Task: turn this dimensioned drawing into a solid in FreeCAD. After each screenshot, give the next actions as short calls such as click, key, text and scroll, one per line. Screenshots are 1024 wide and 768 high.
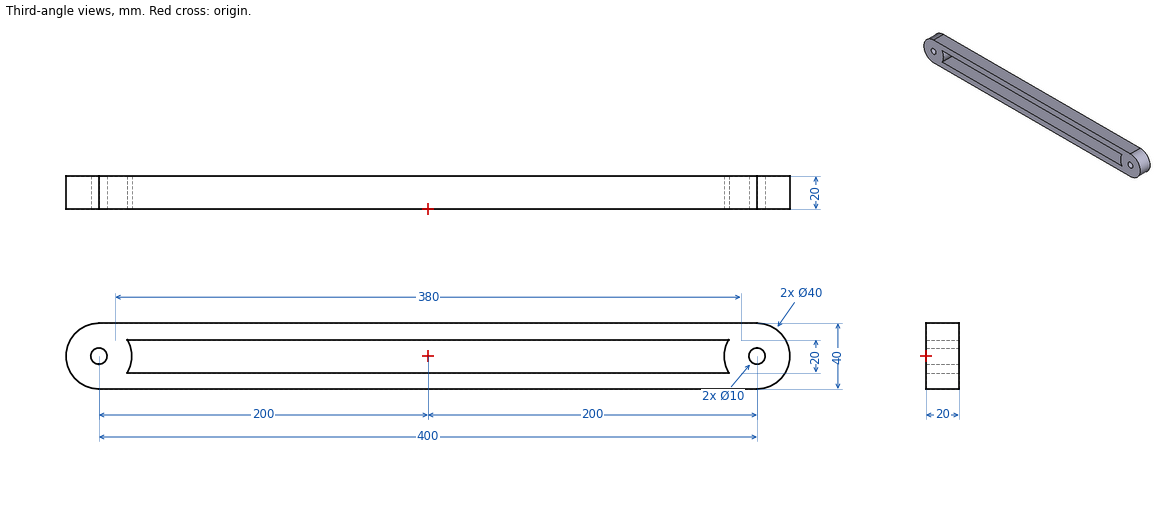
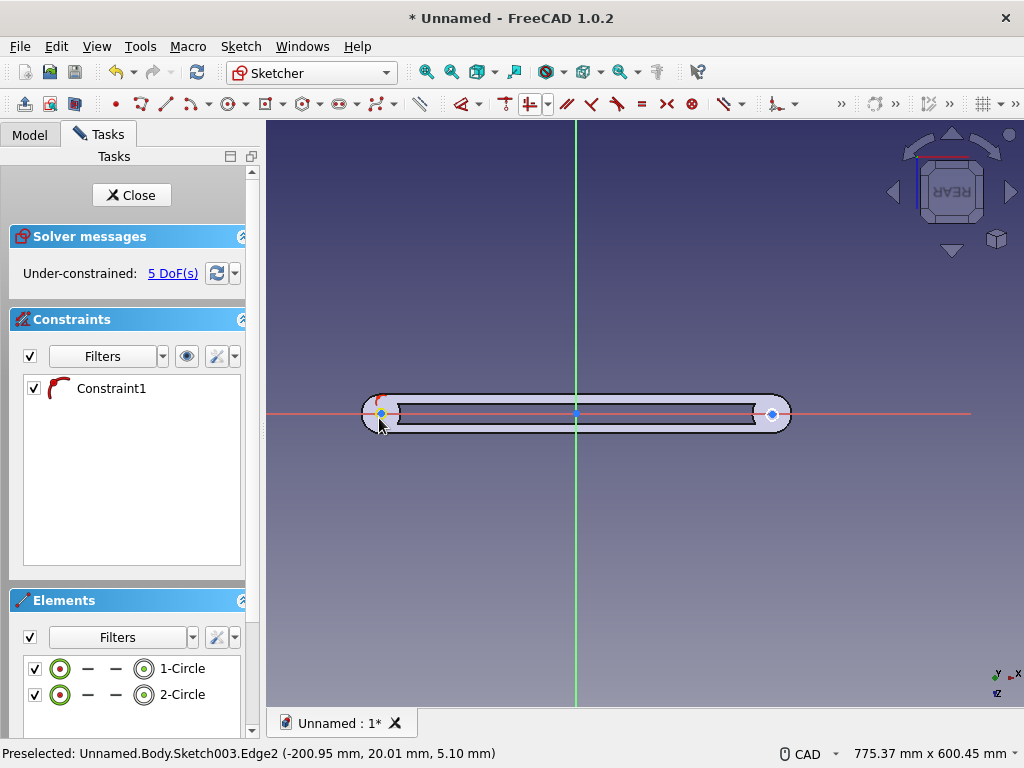
scroll(776, 411, up, 8)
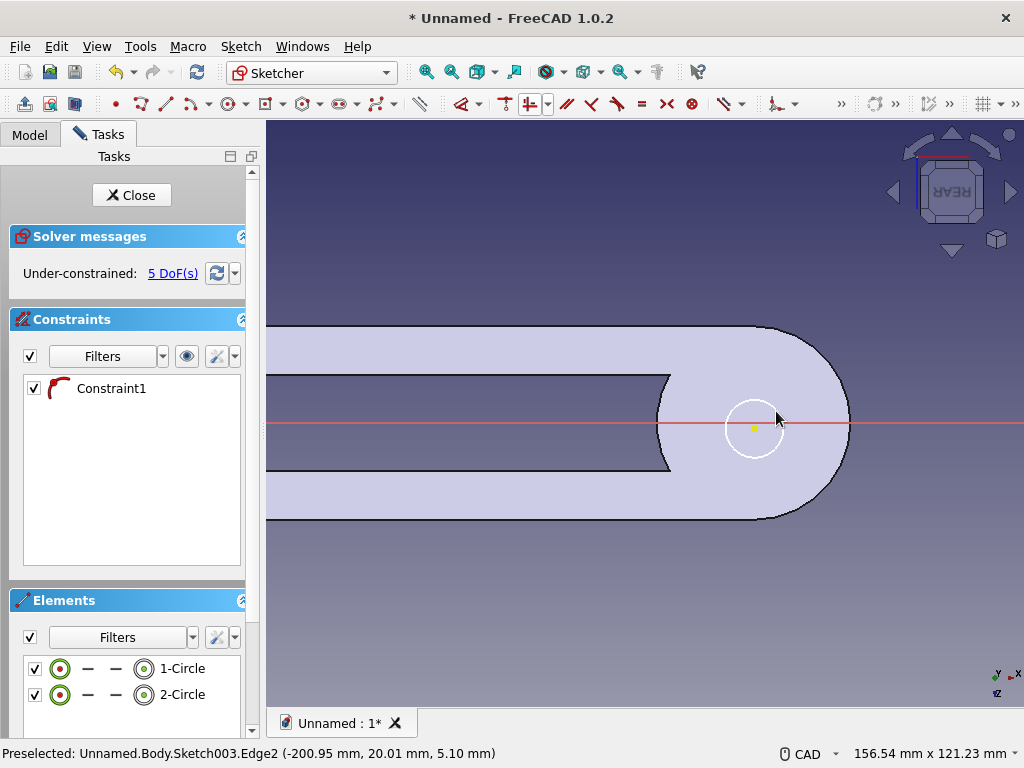
click(775, 408)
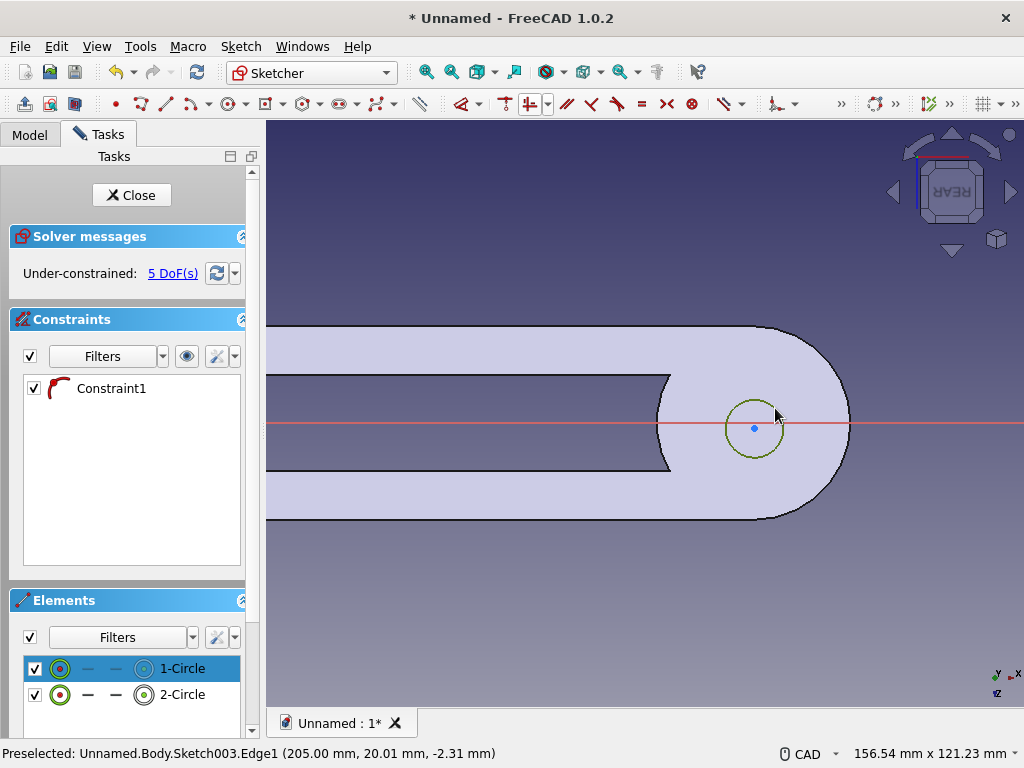
scroll(777, 411, down, 8)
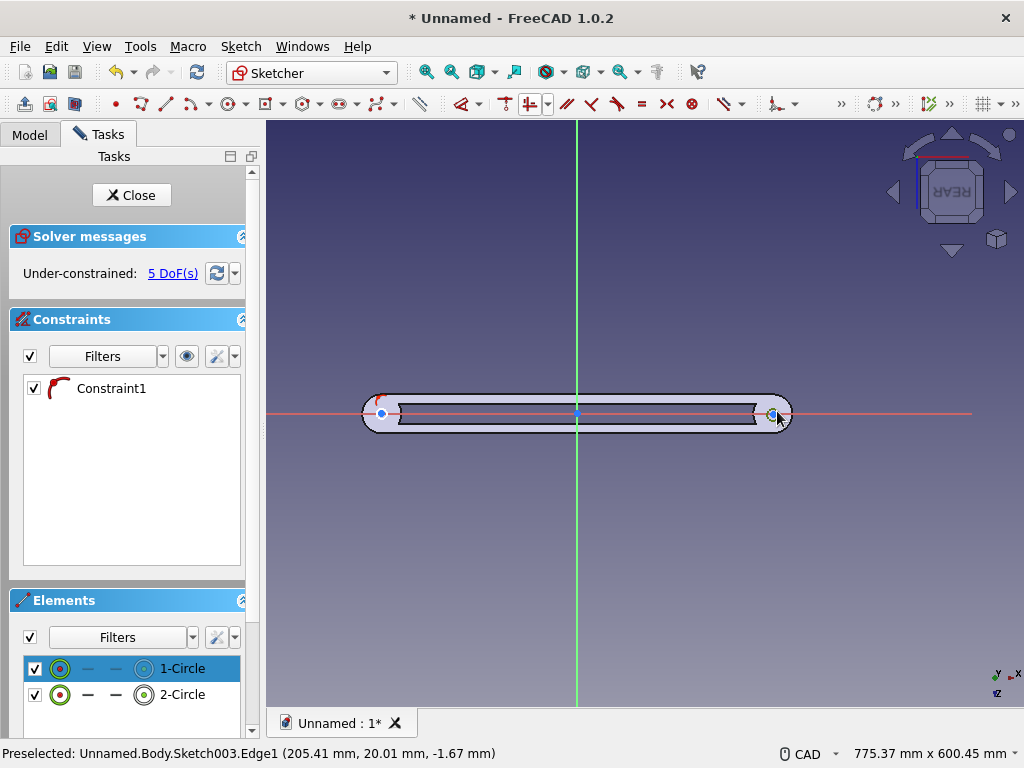
scroll(385, 410, up, 7)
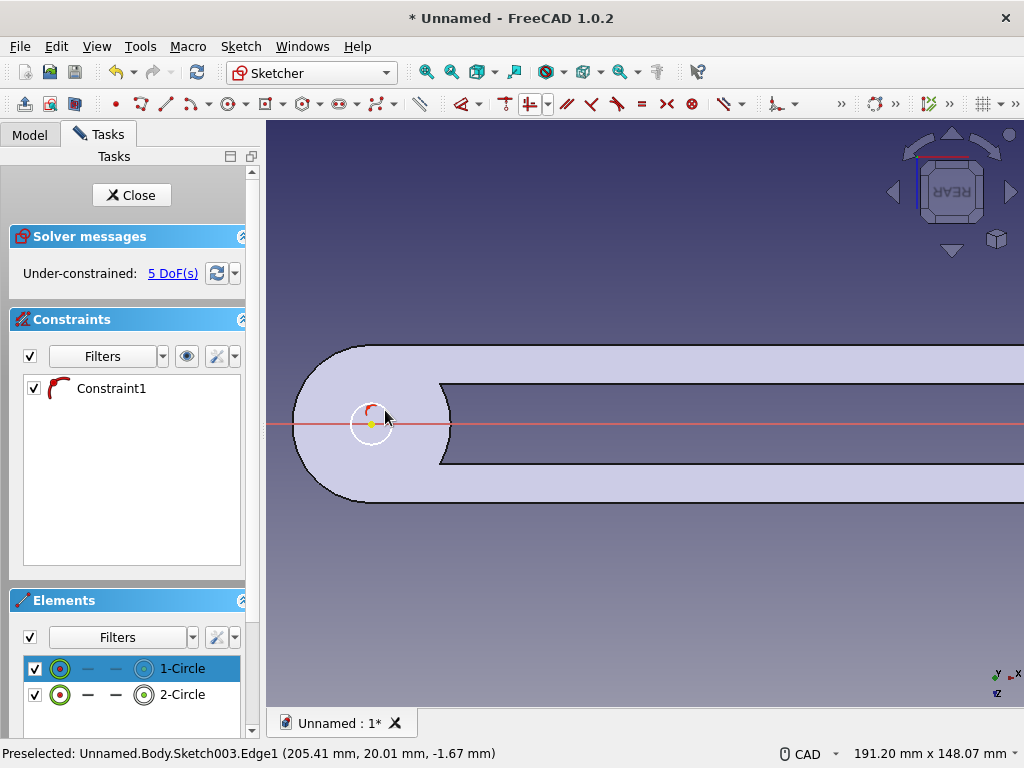
click(386, 409)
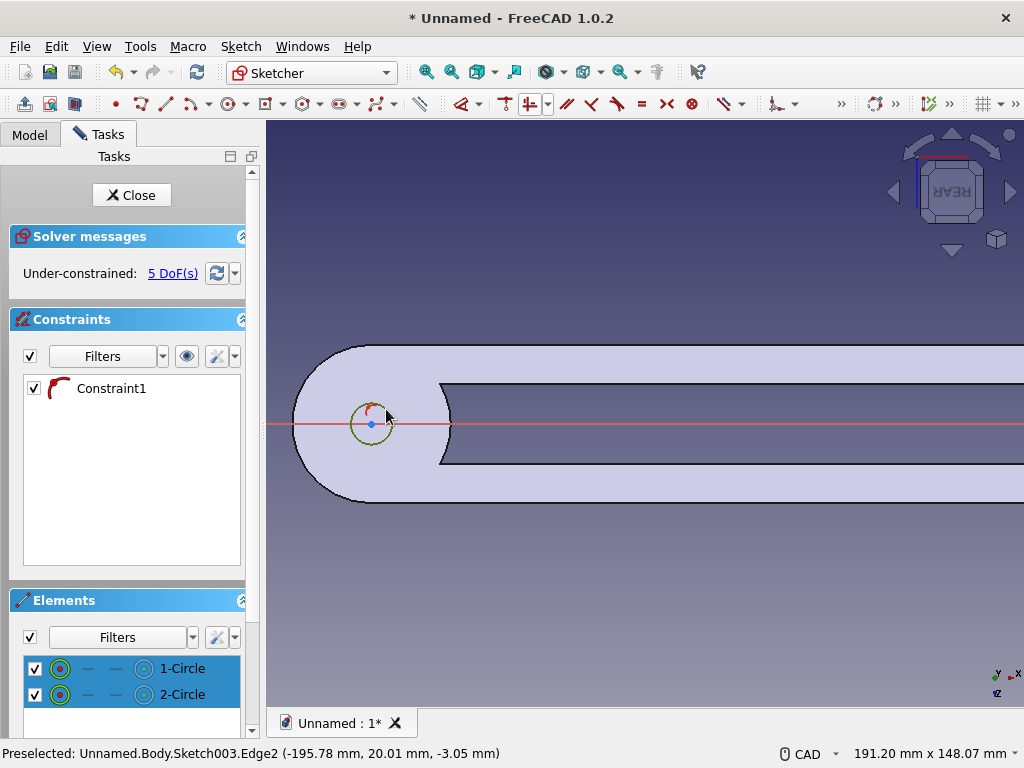
click(642, 104)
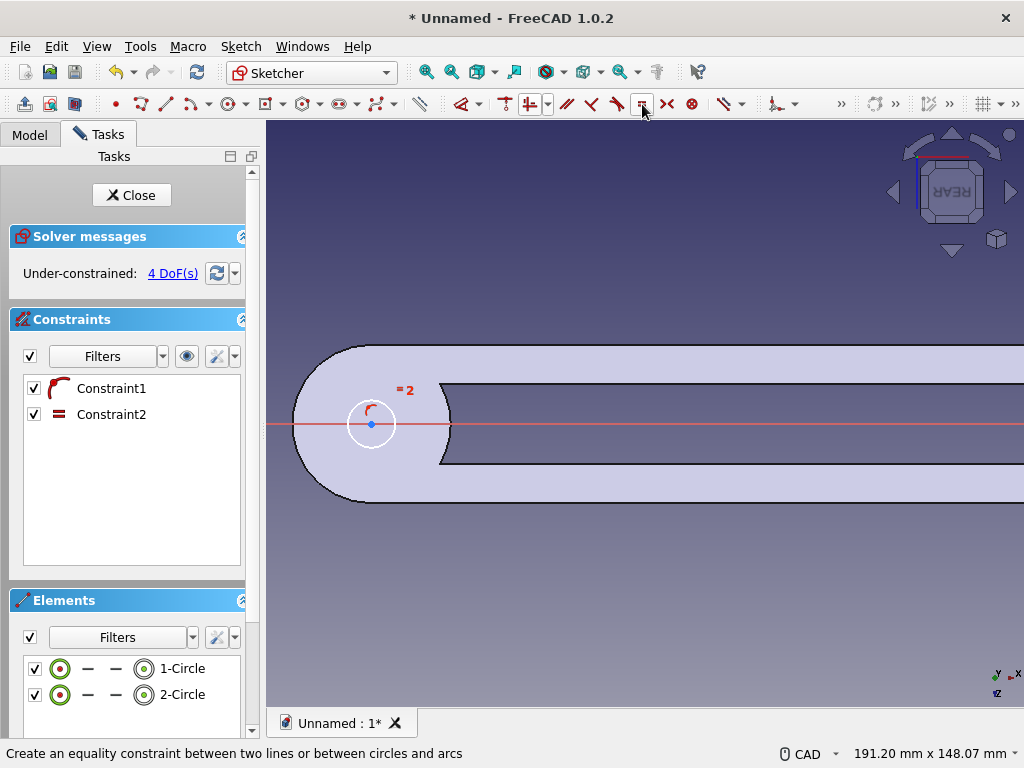
scroll(384, 410, down, 7)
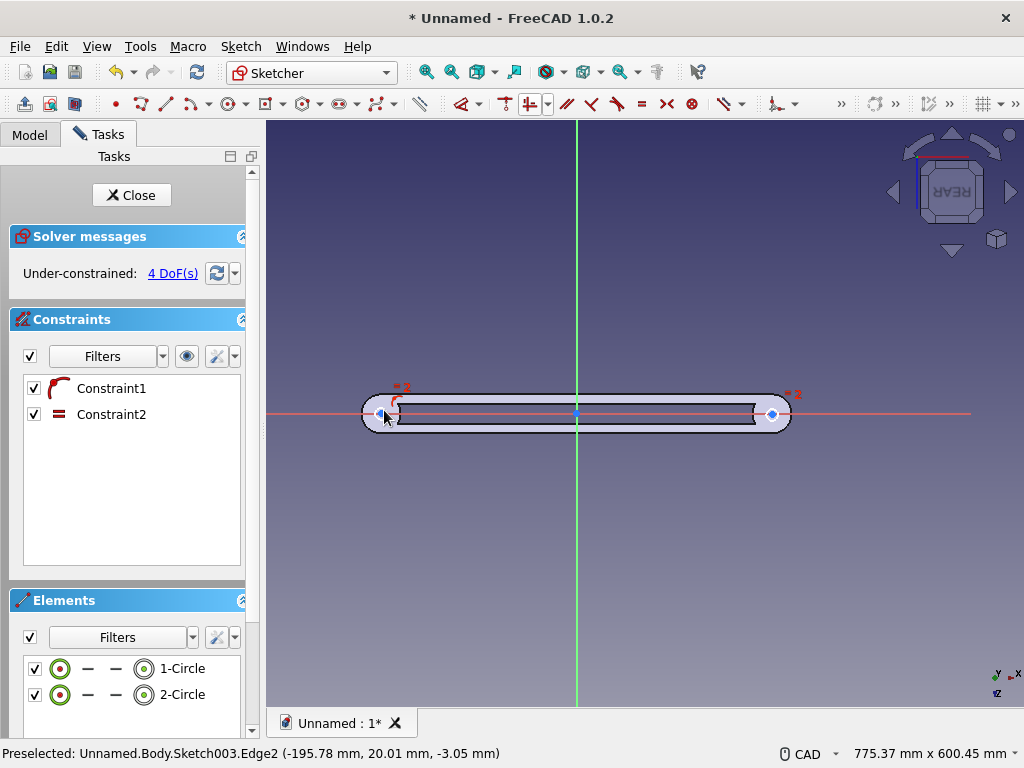
click(772, 415)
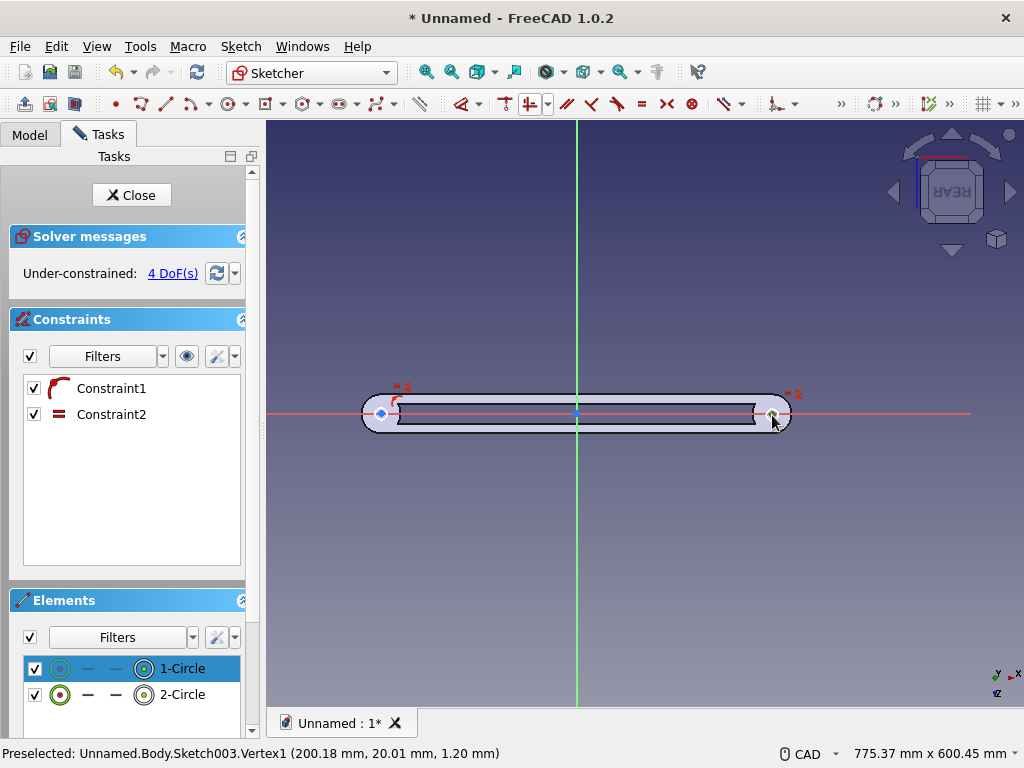
click(334, 414)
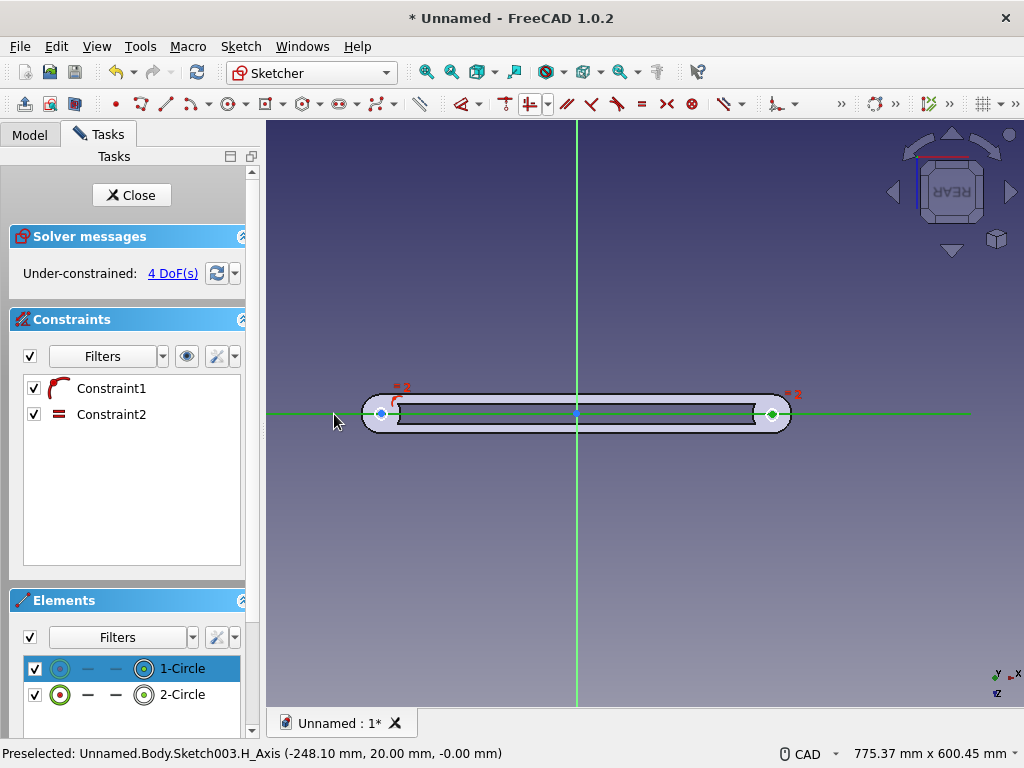
click(505, 104)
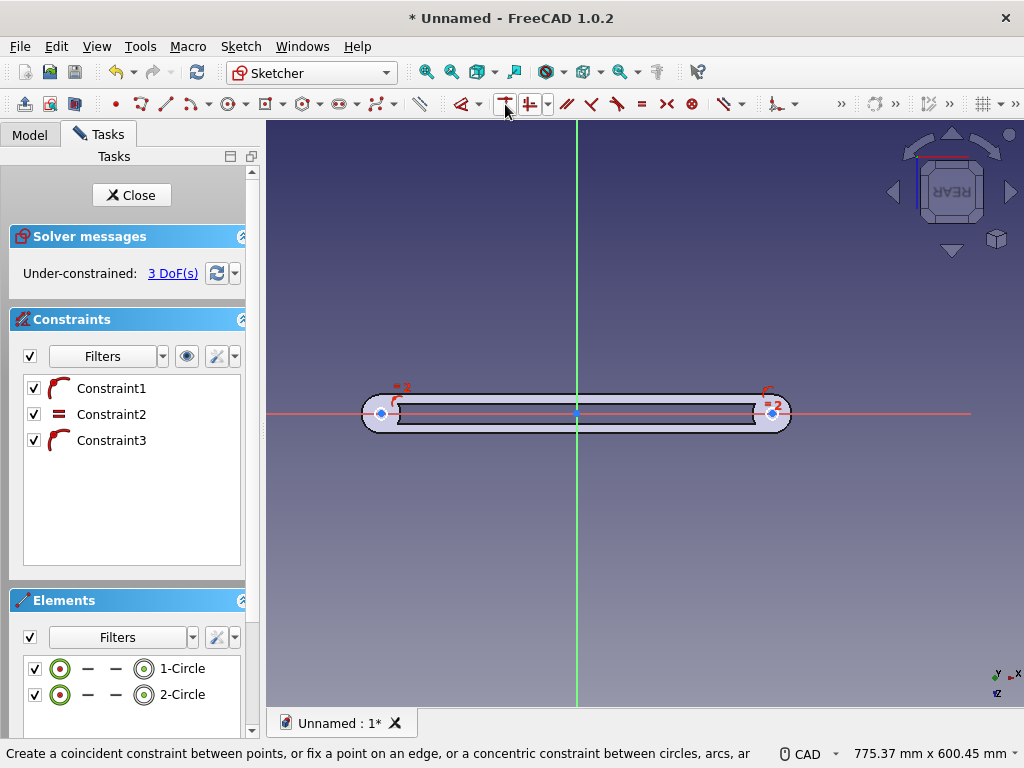
click(460, 104)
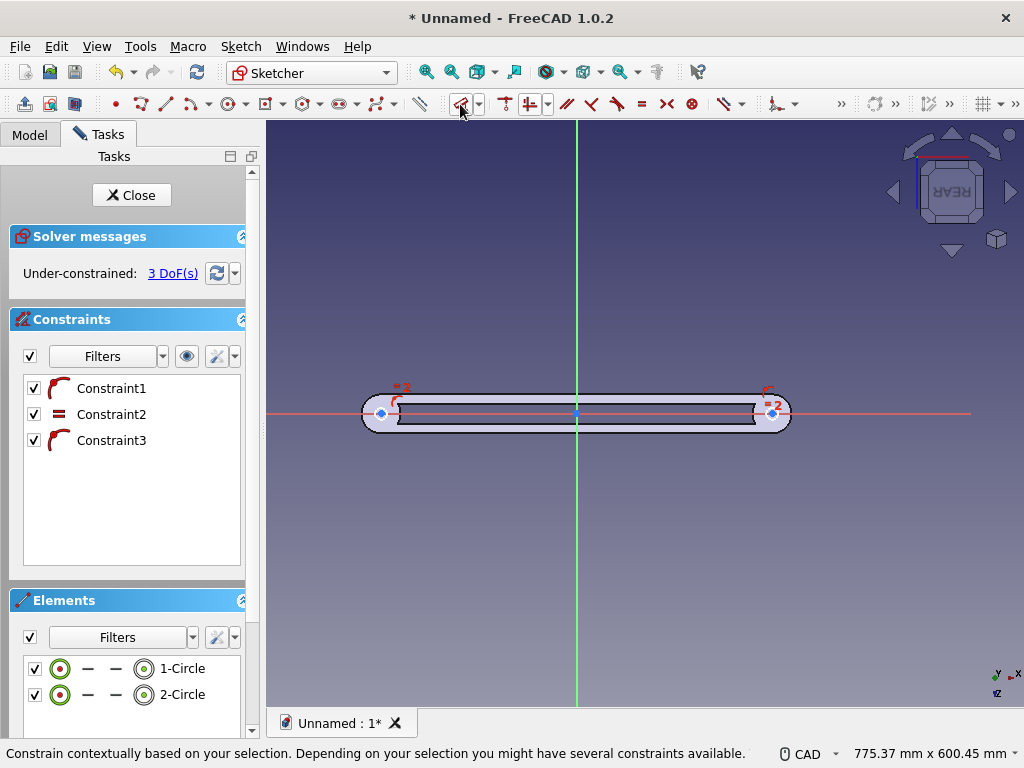
scroll(766, 414, up, 8)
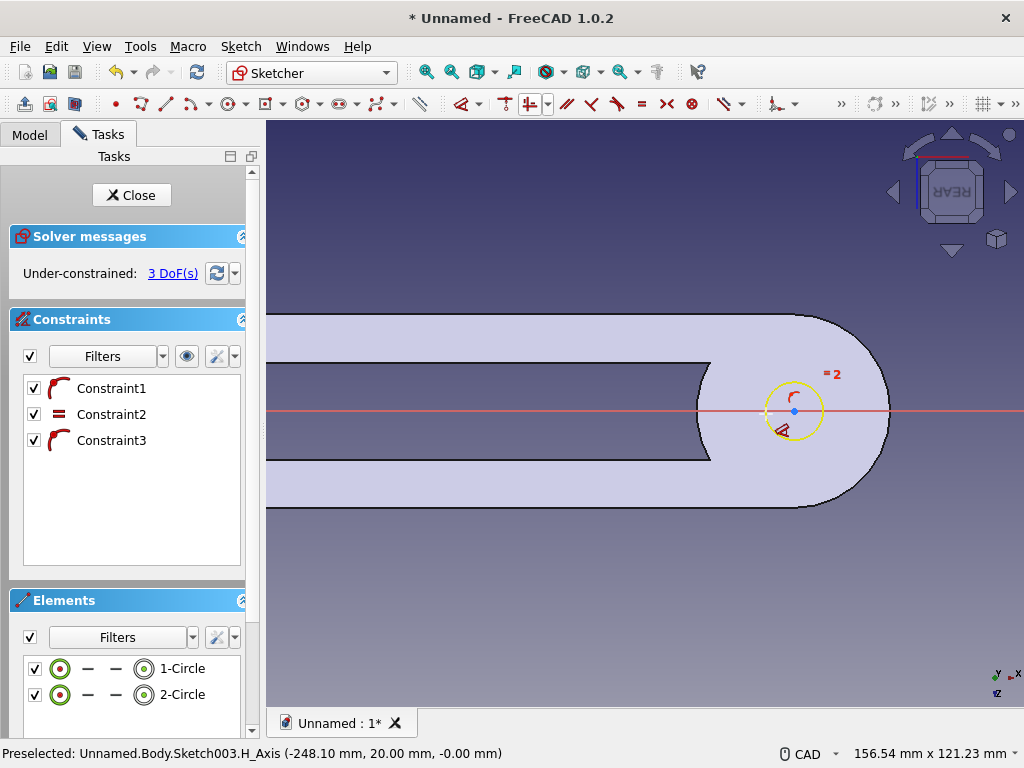
click(765, 410)
click(742, 380)